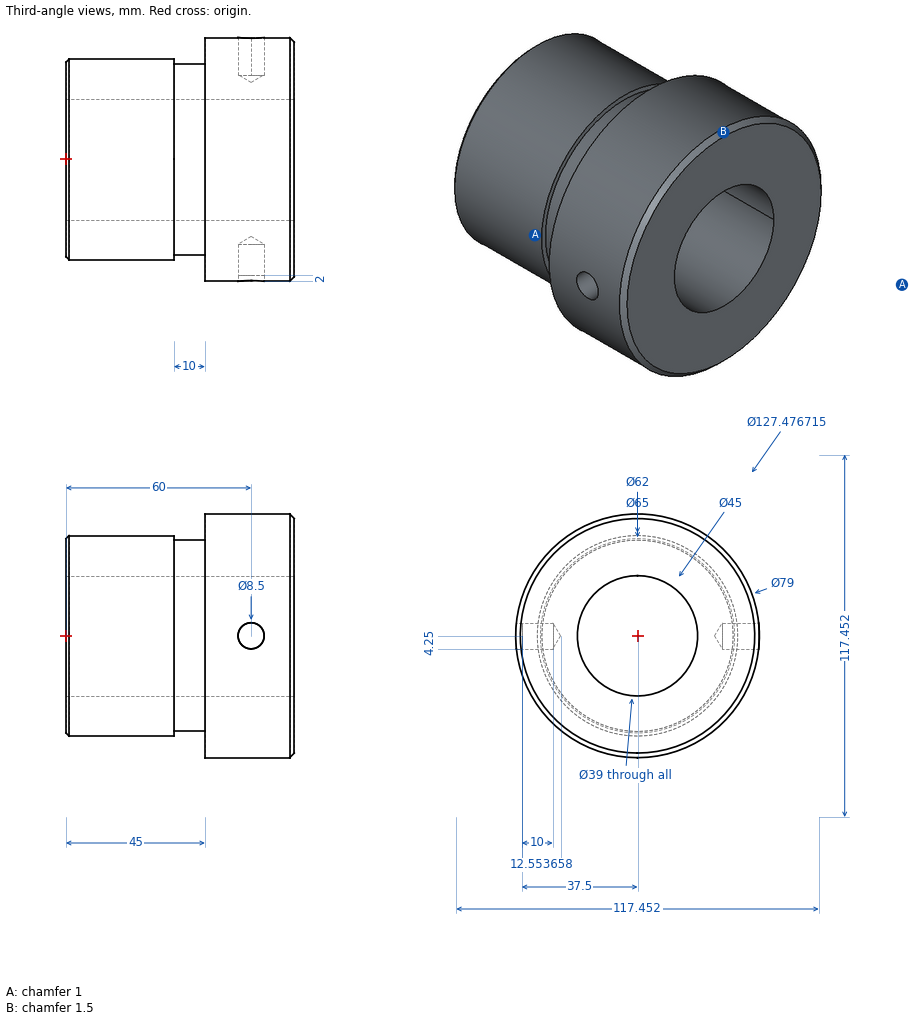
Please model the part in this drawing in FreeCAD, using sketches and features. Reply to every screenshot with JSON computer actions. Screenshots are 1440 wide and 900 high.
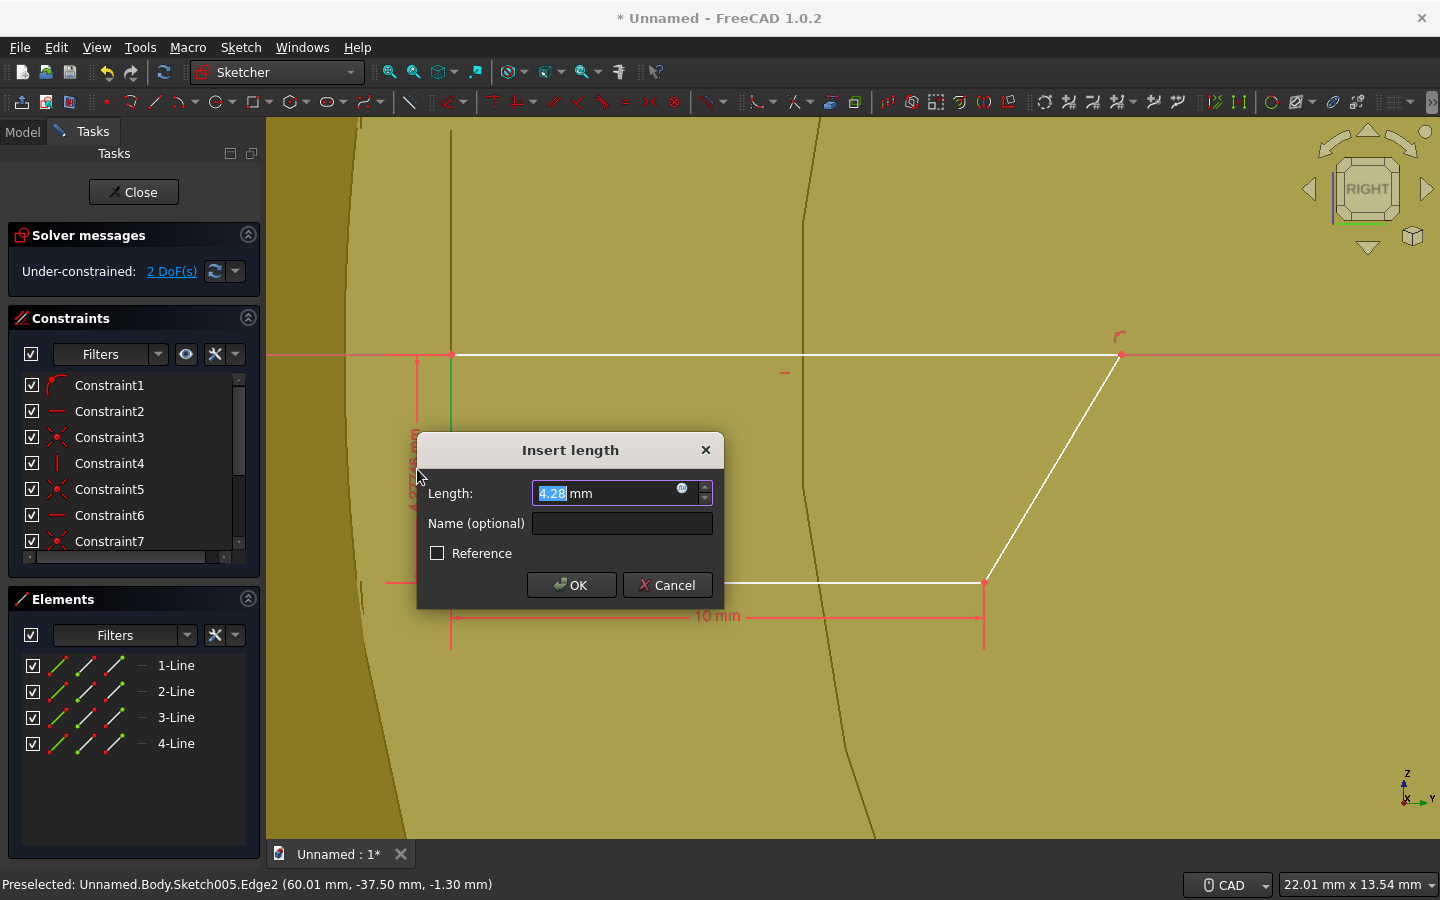
{"action": "type", "text": "4.25"}
{"action": "key", "text": "Return"}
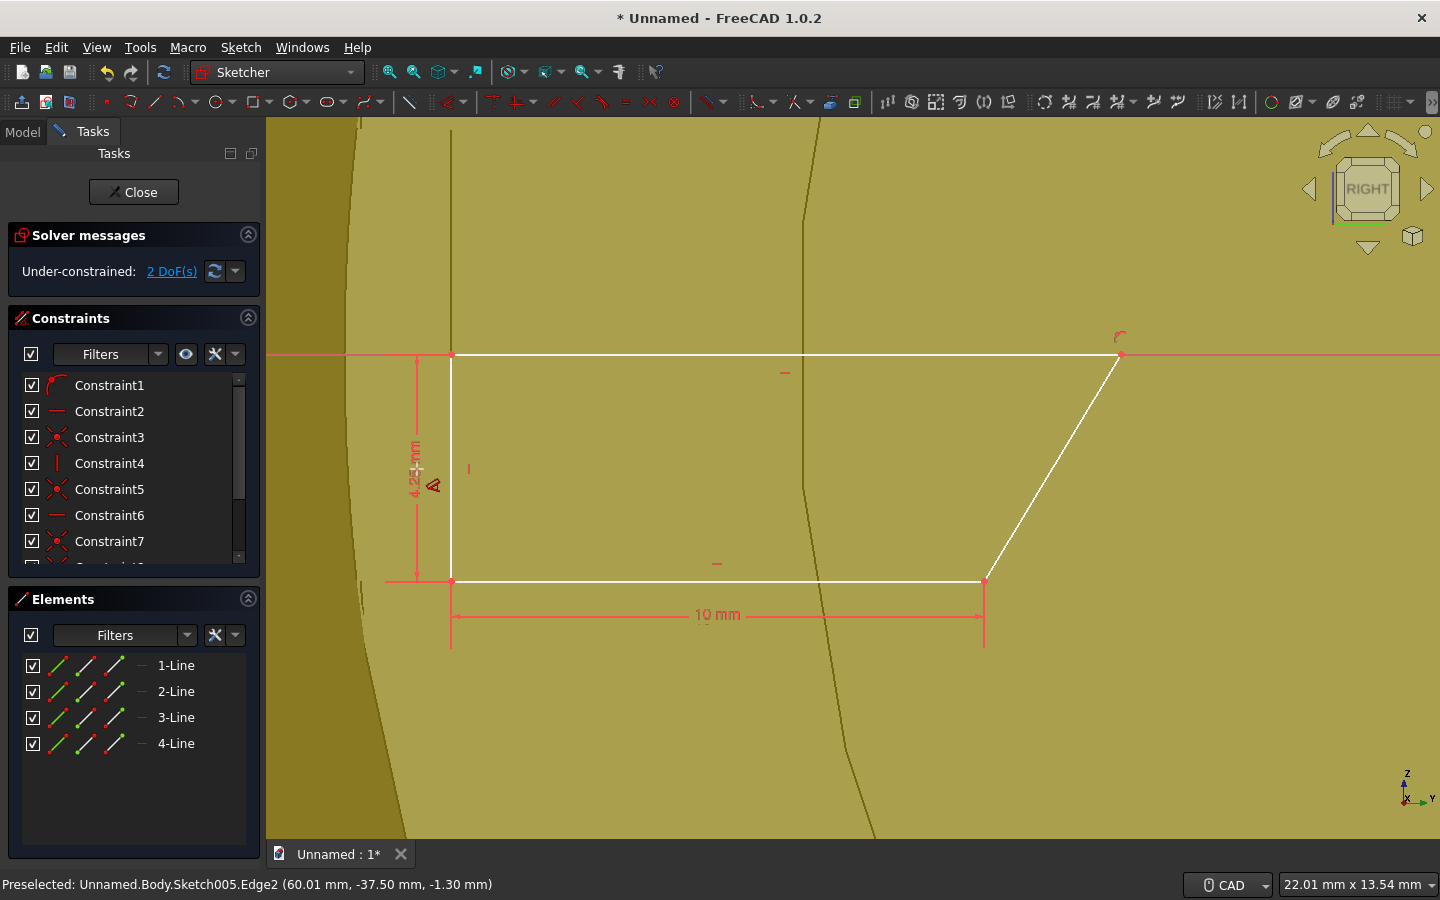
{"action": "left_click", "coordinate": [451, 355]}
{"action": "left_click", "coordinate": [863, 321]}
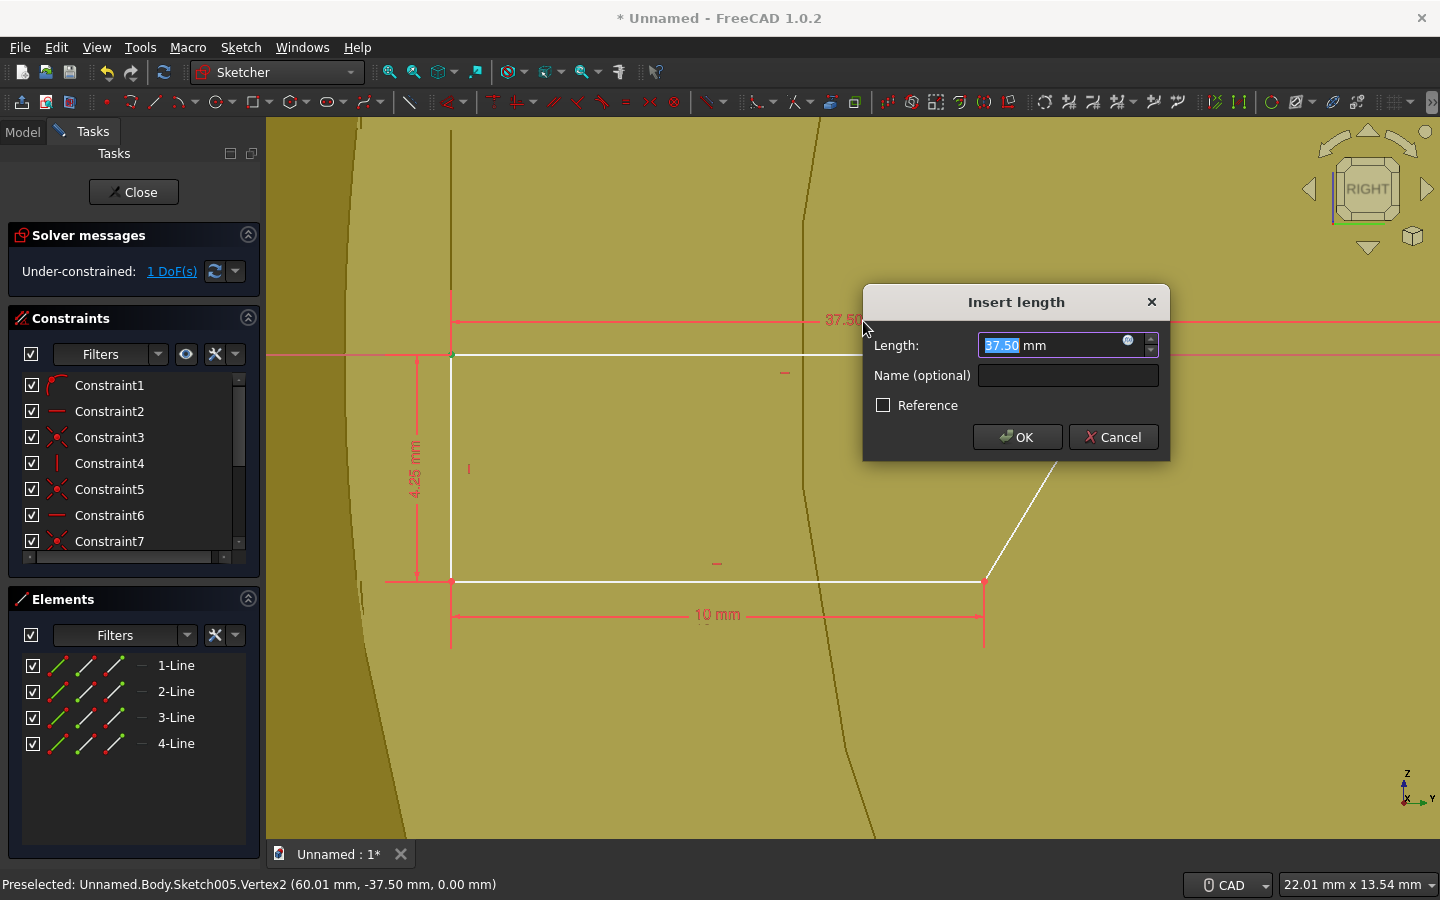
{"action": "type", "text": "37.5"}
{"action": "key", "text": "Return"}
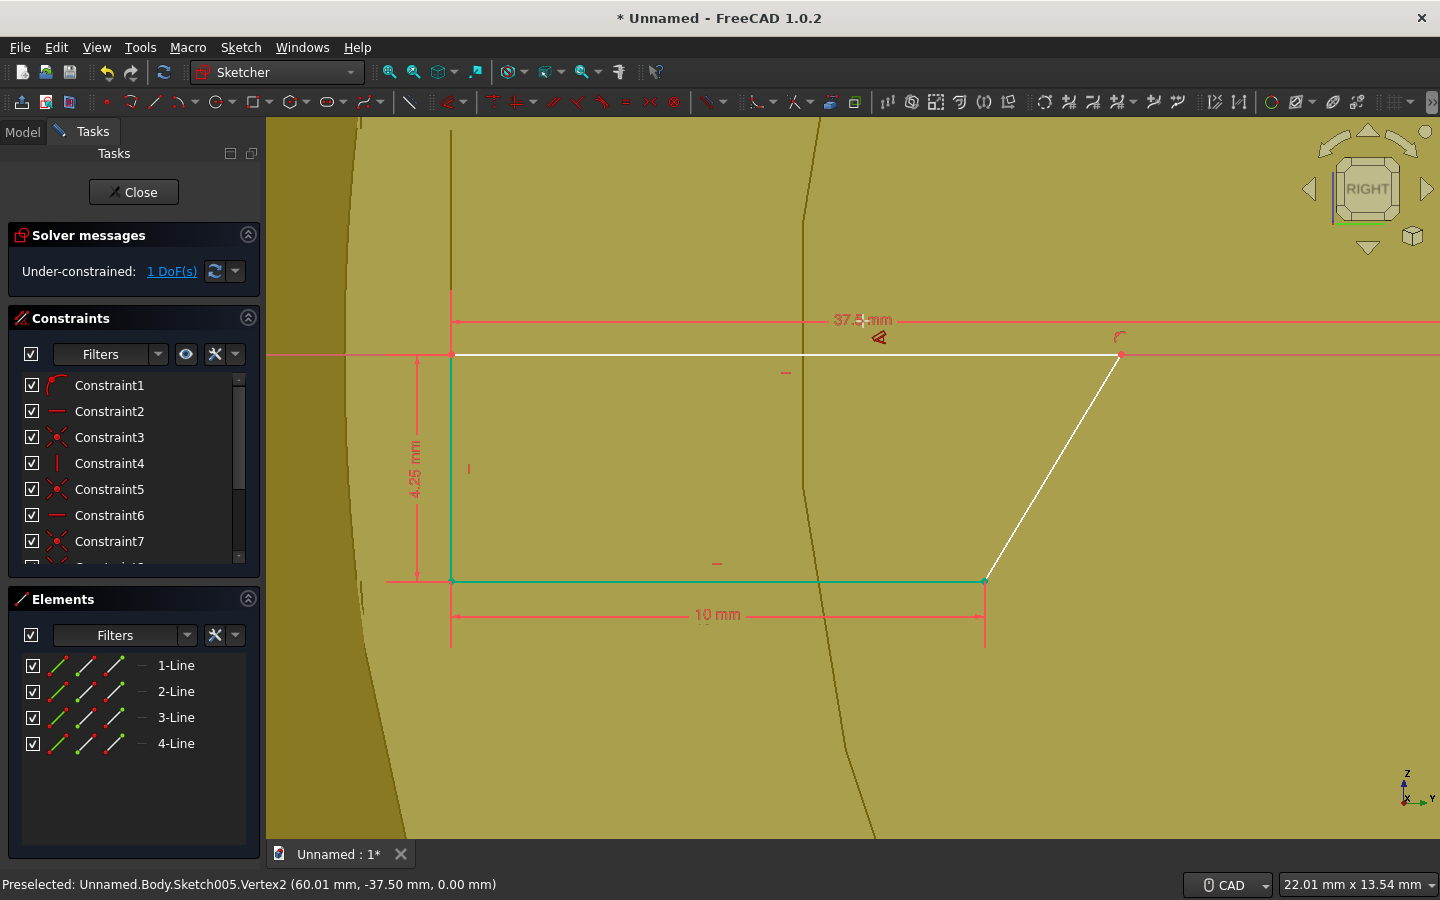
{"action": "left_click", "coordinate": [920, 355]}
{"action": "left_click", "coordinate": [786, 321]}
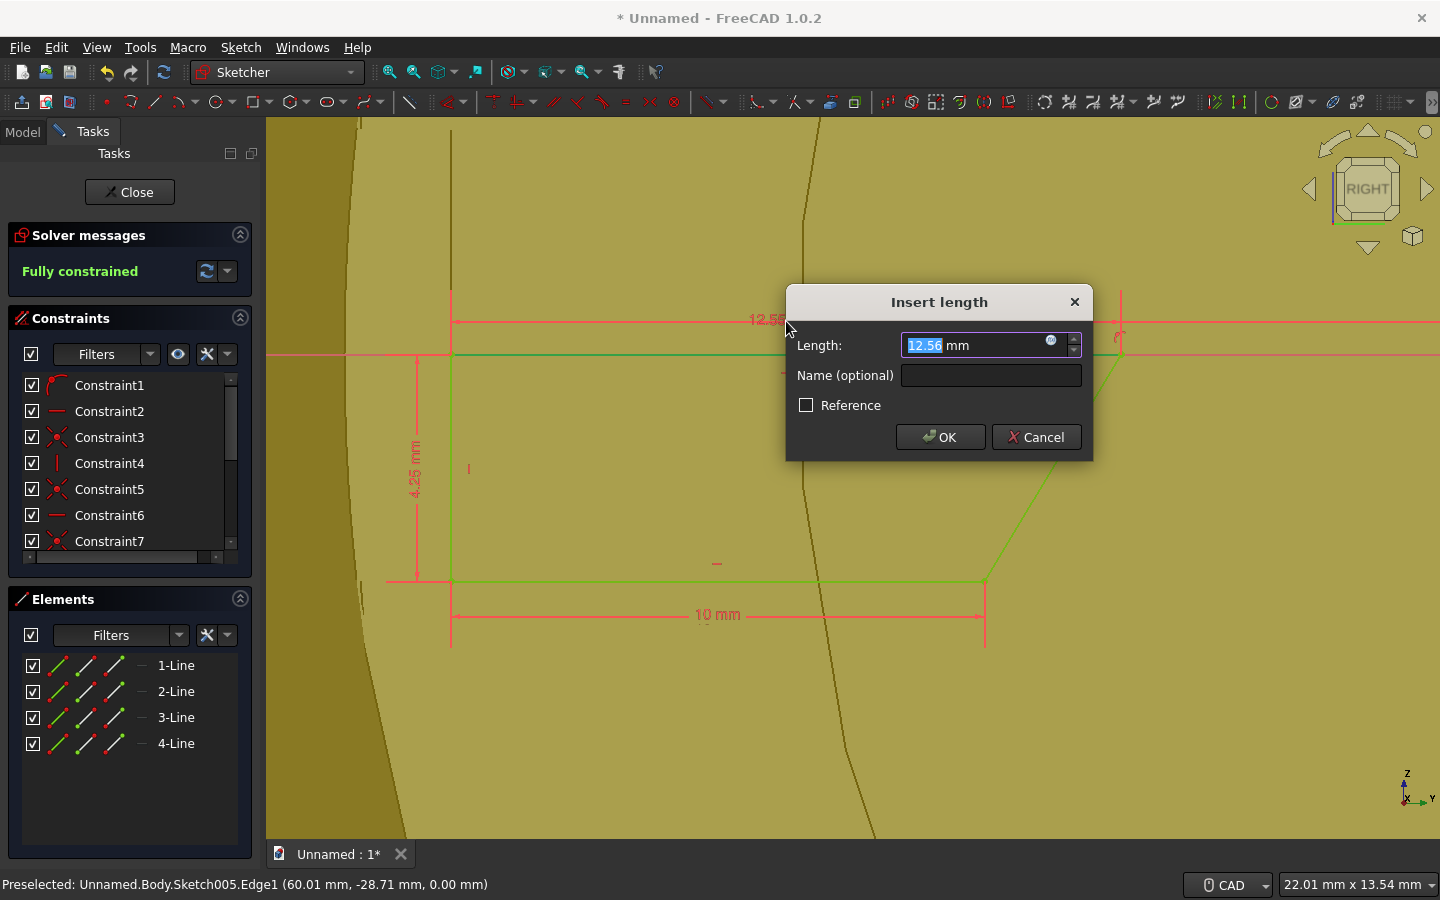
{"action": "type", "text": "12.553658"}
{"action": "key", "text": "Return"}
{"action": "key", "text": "Escape"}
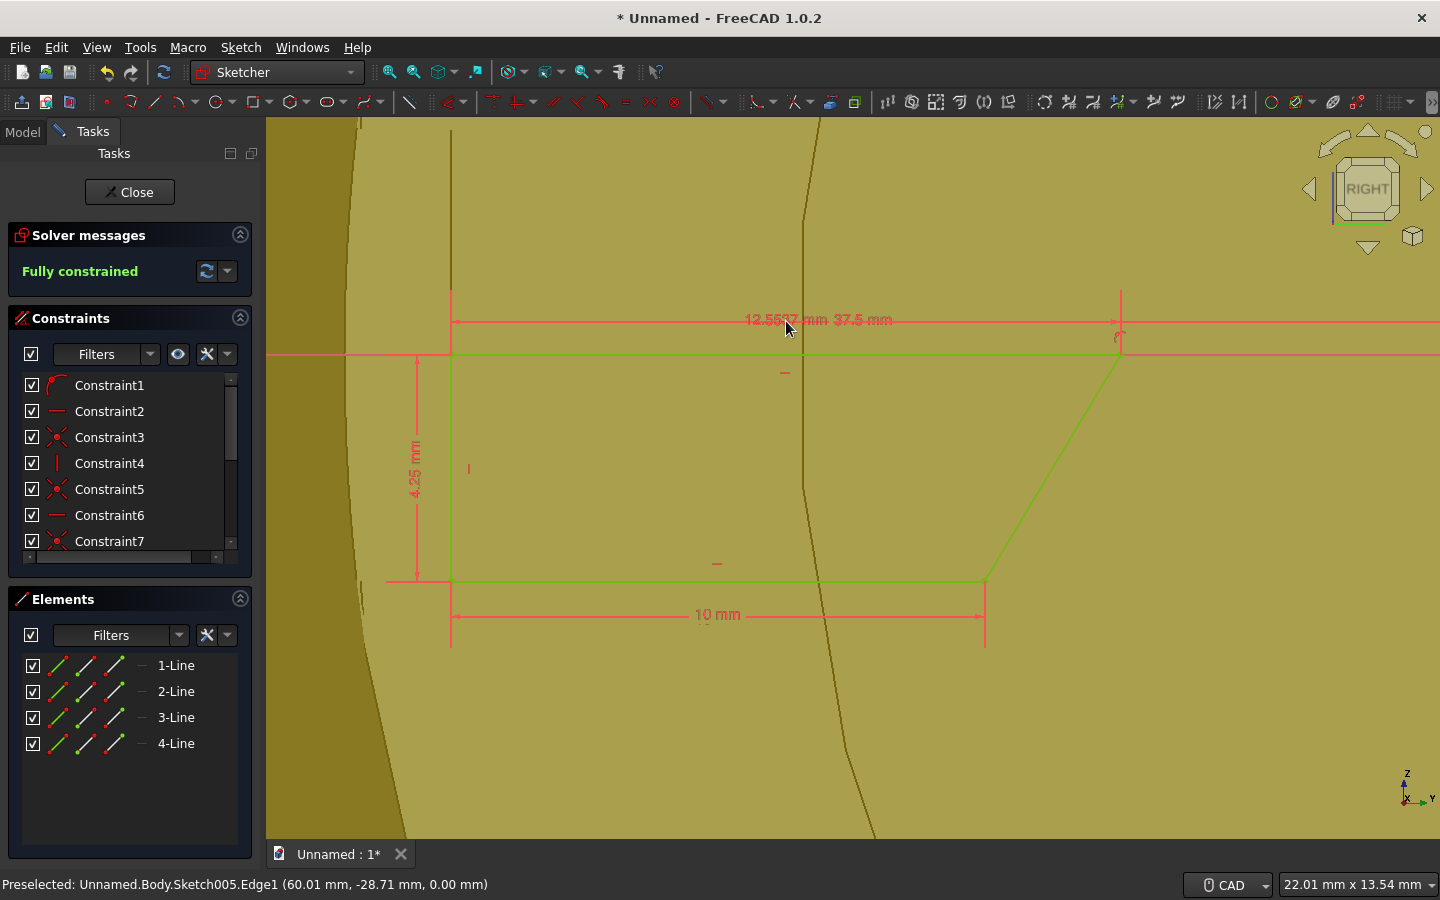
{"action": "left_click", "coordinate": [130, 192]}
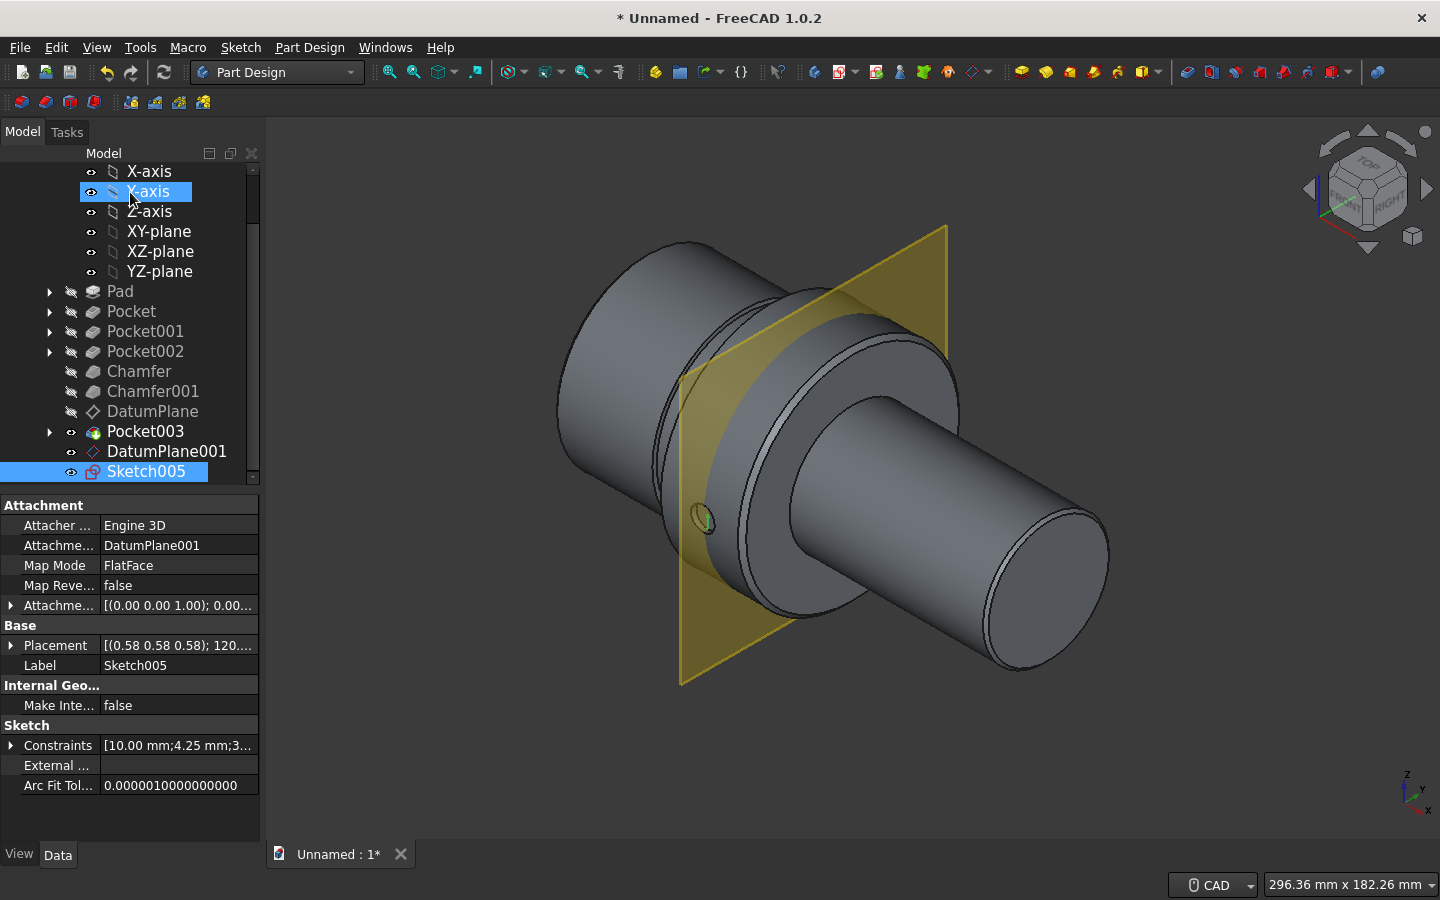
{"action": "left_click", "coordinate": [1236, 72]}